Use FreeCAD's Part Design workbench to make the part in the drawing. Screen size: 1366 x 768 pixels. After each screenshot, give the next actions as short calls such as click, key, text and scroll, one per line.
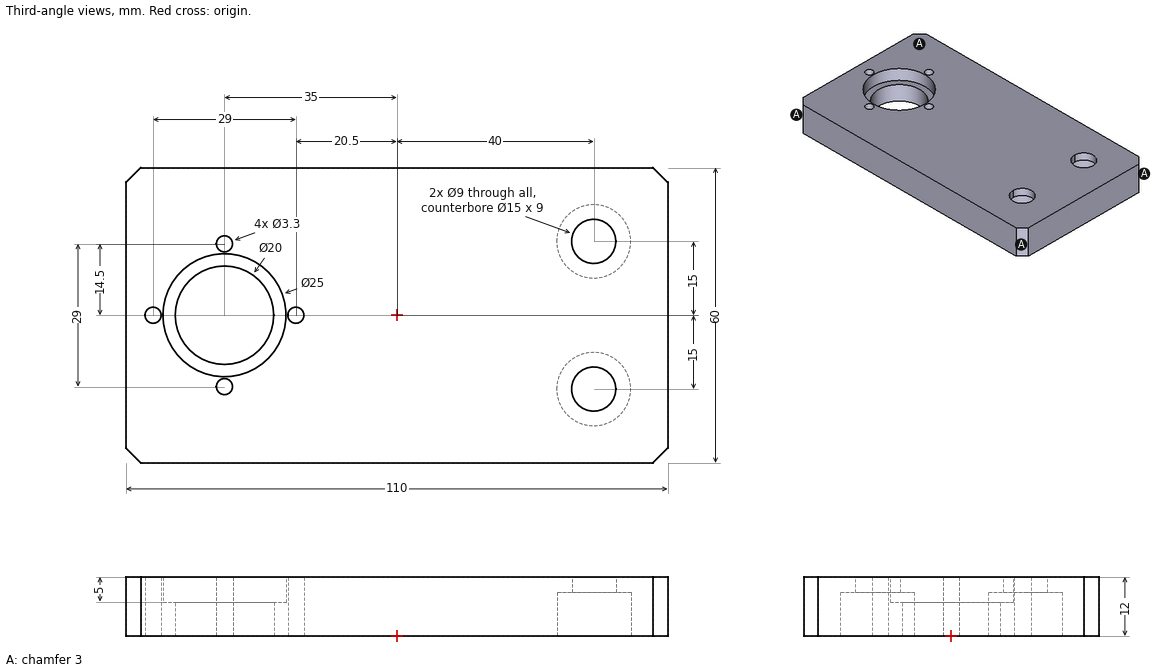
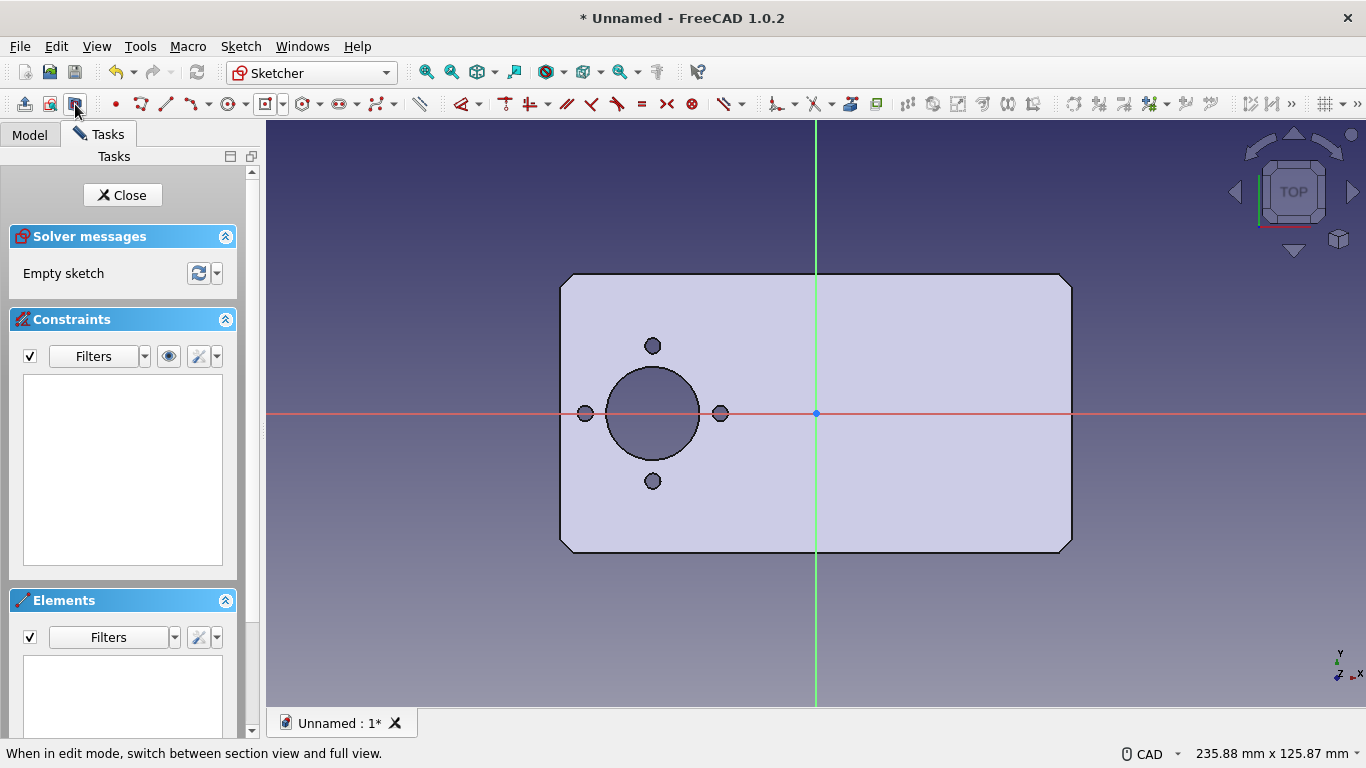
scroll(1060, 413, up, 4)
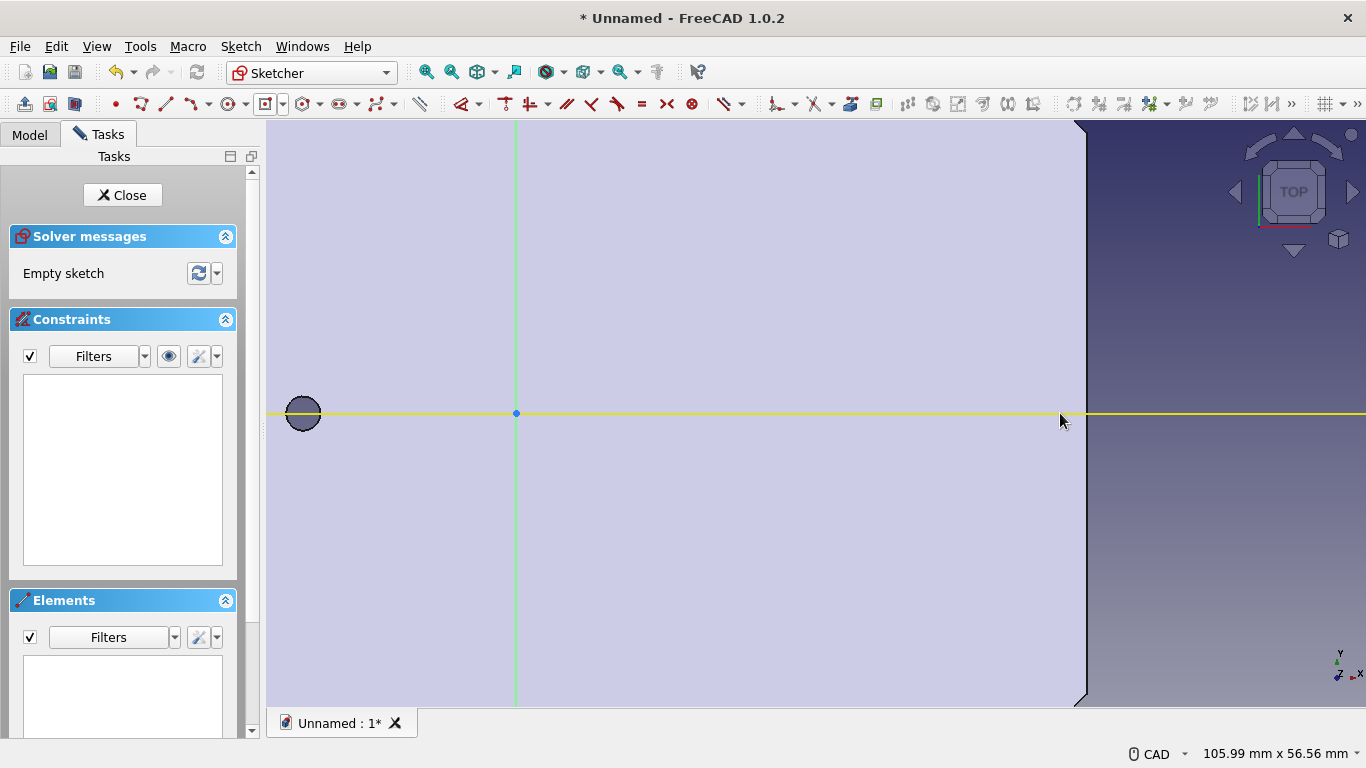
key(g)
key(c)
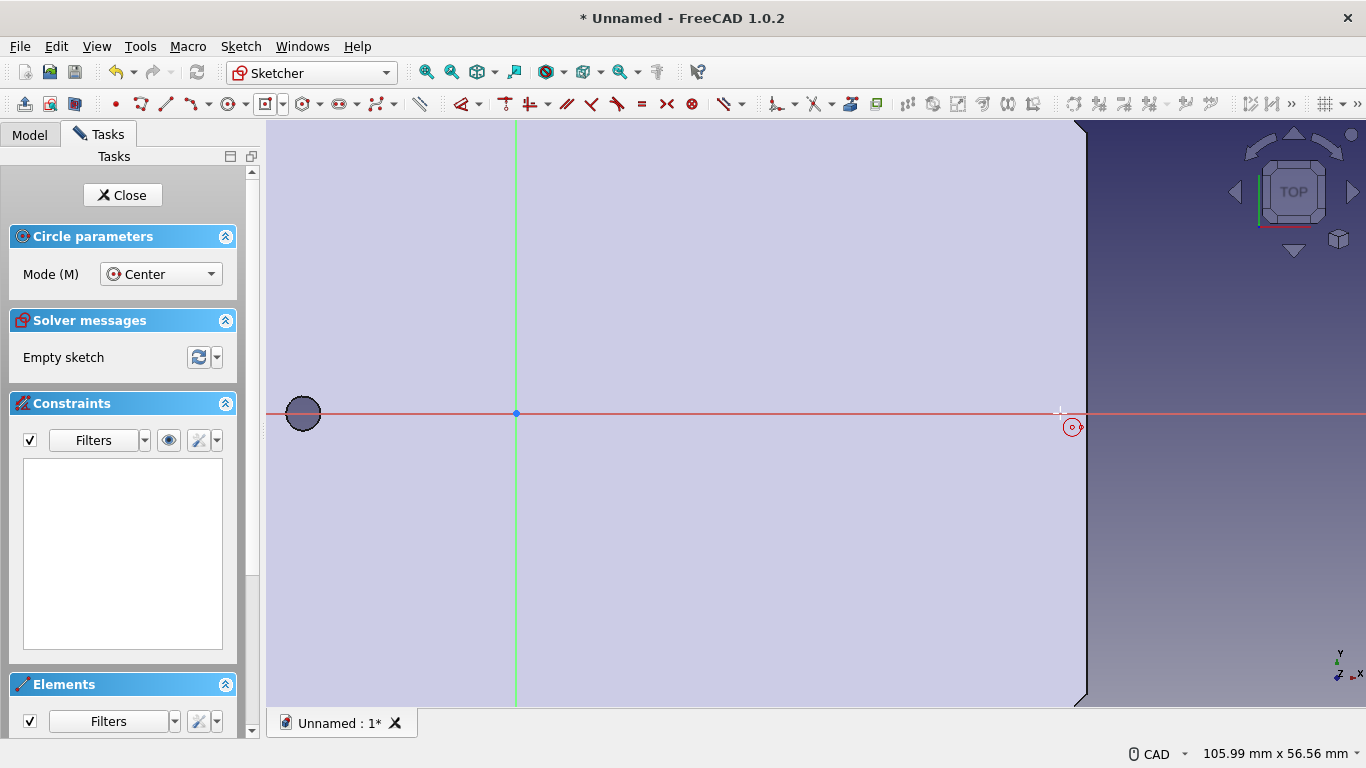
click(931, 258)
click(964, 225)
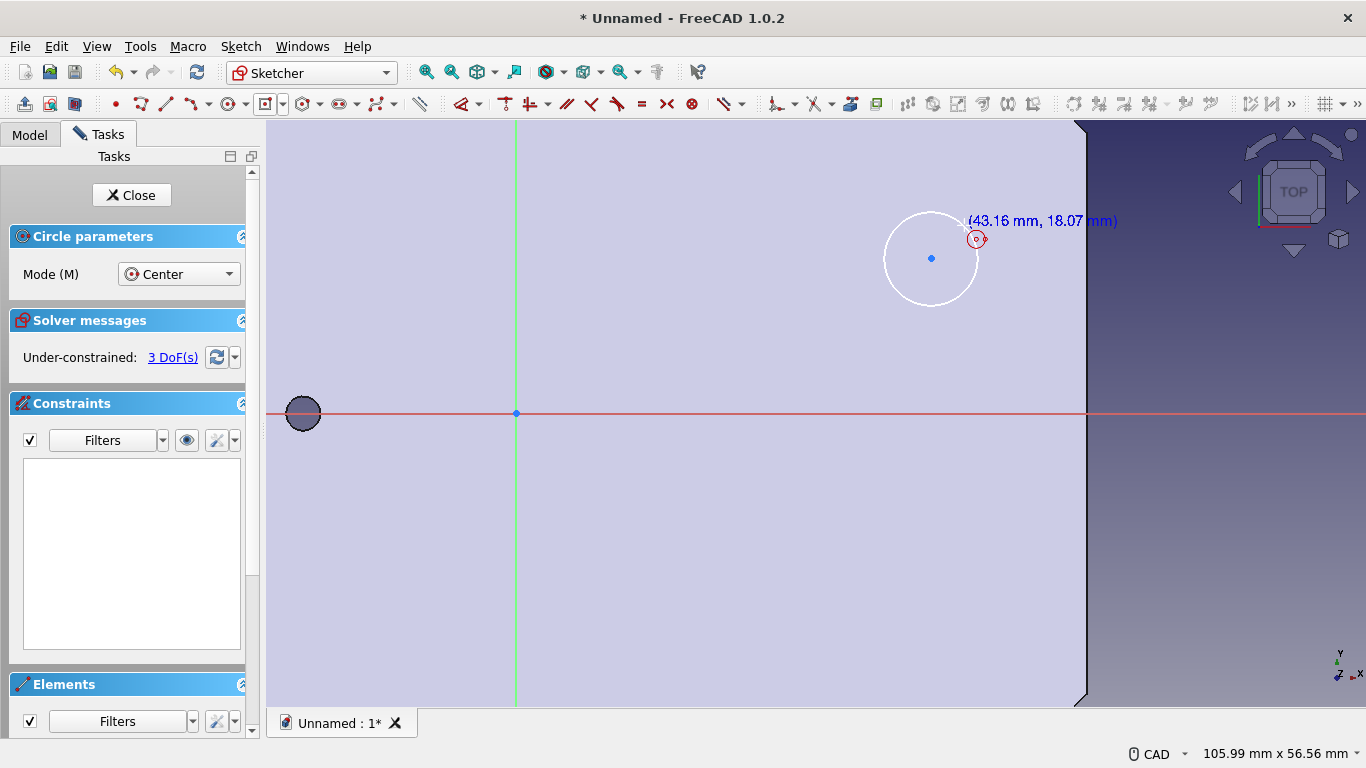
click(931, 569)
click(964, 536)
key(Escape)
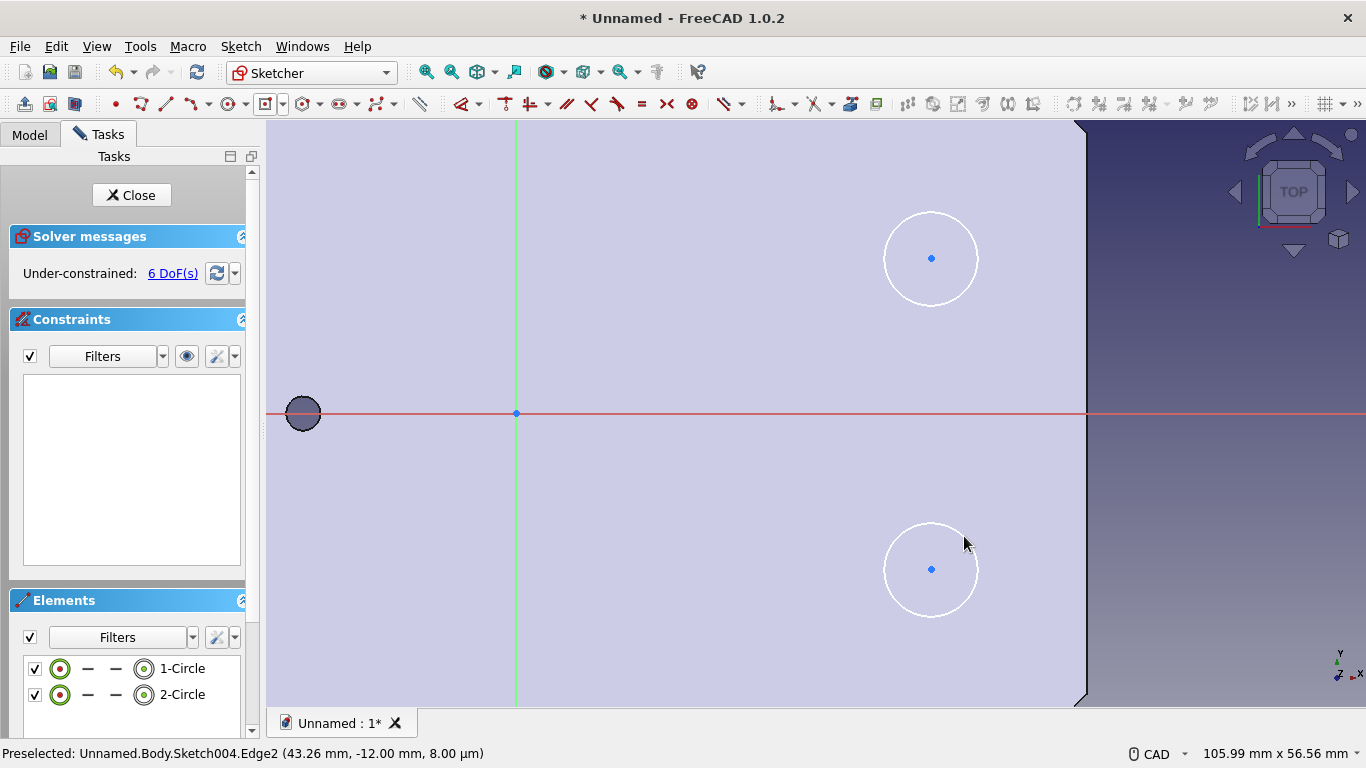
click(964, 226)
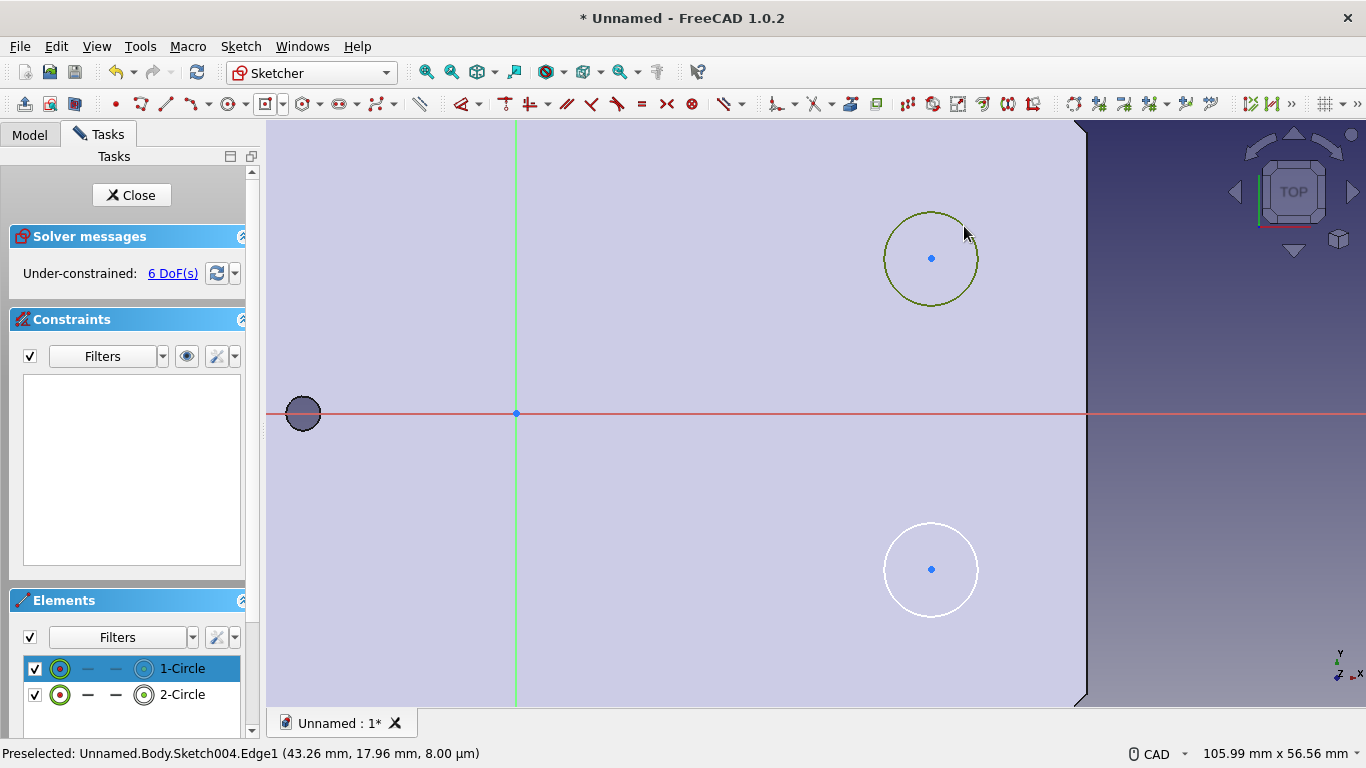
click(964, 537)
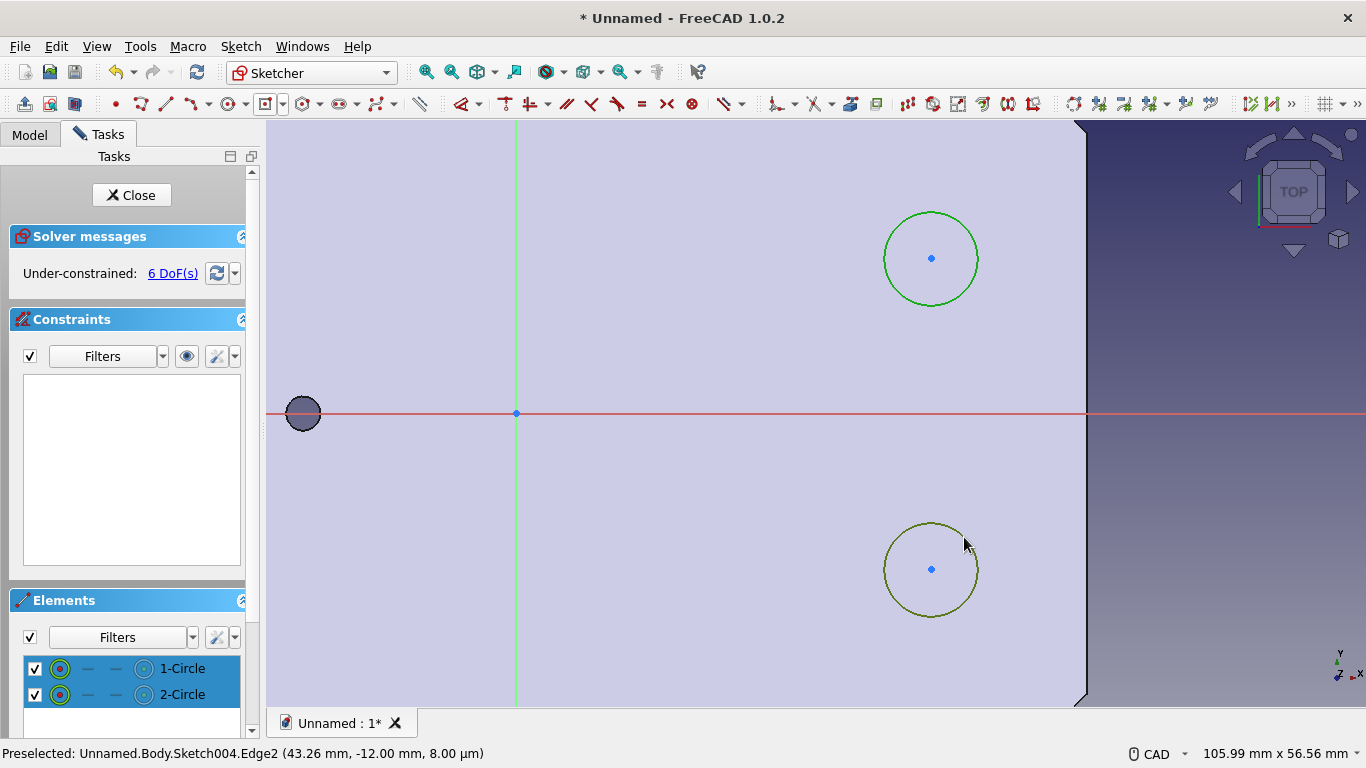
click(642, 104)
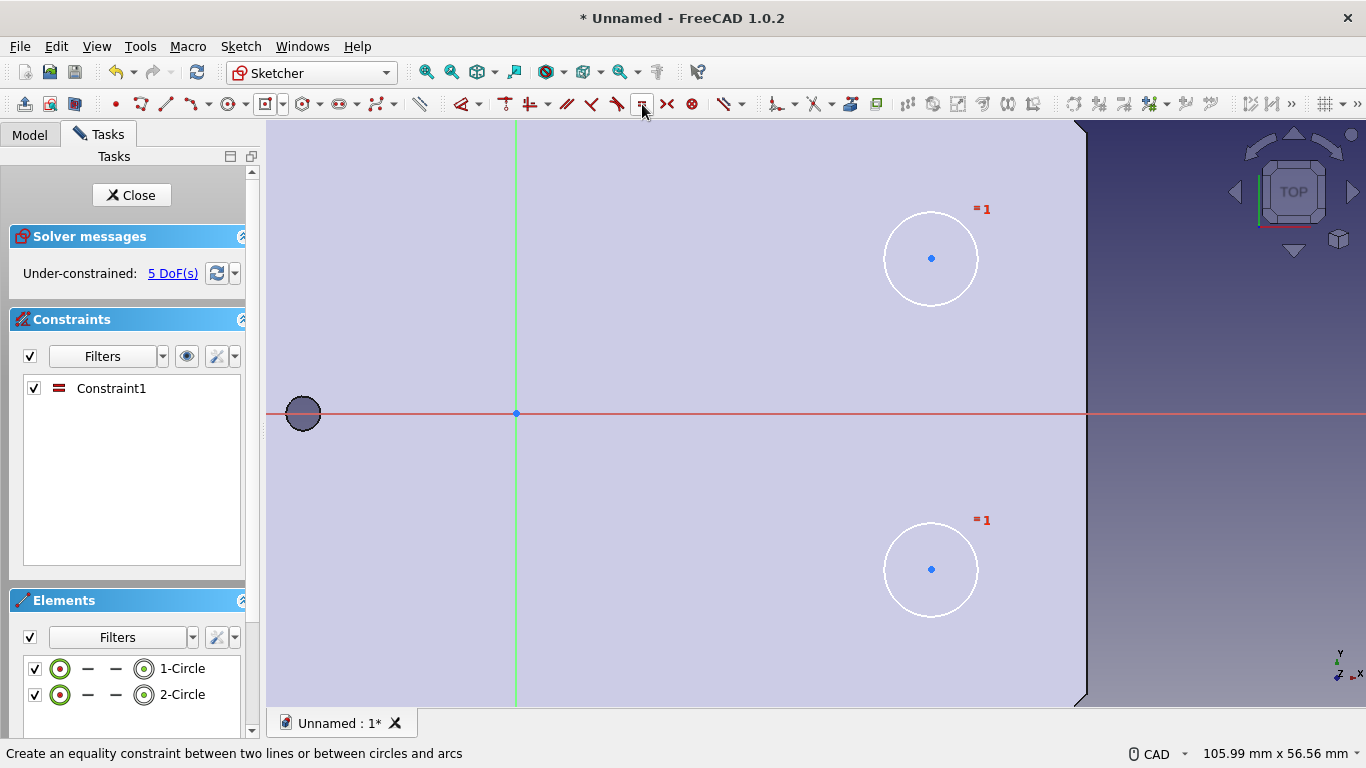
click(931, 259)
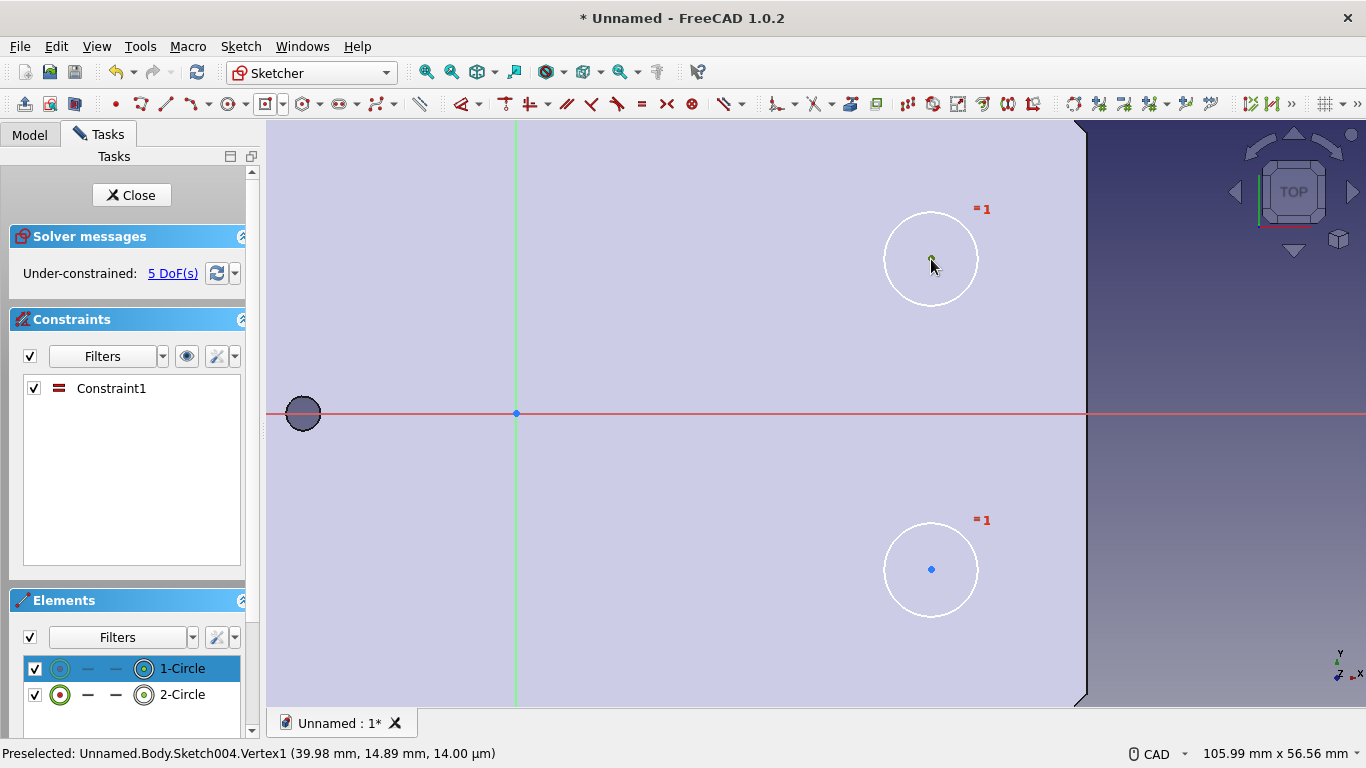
click(931, 570)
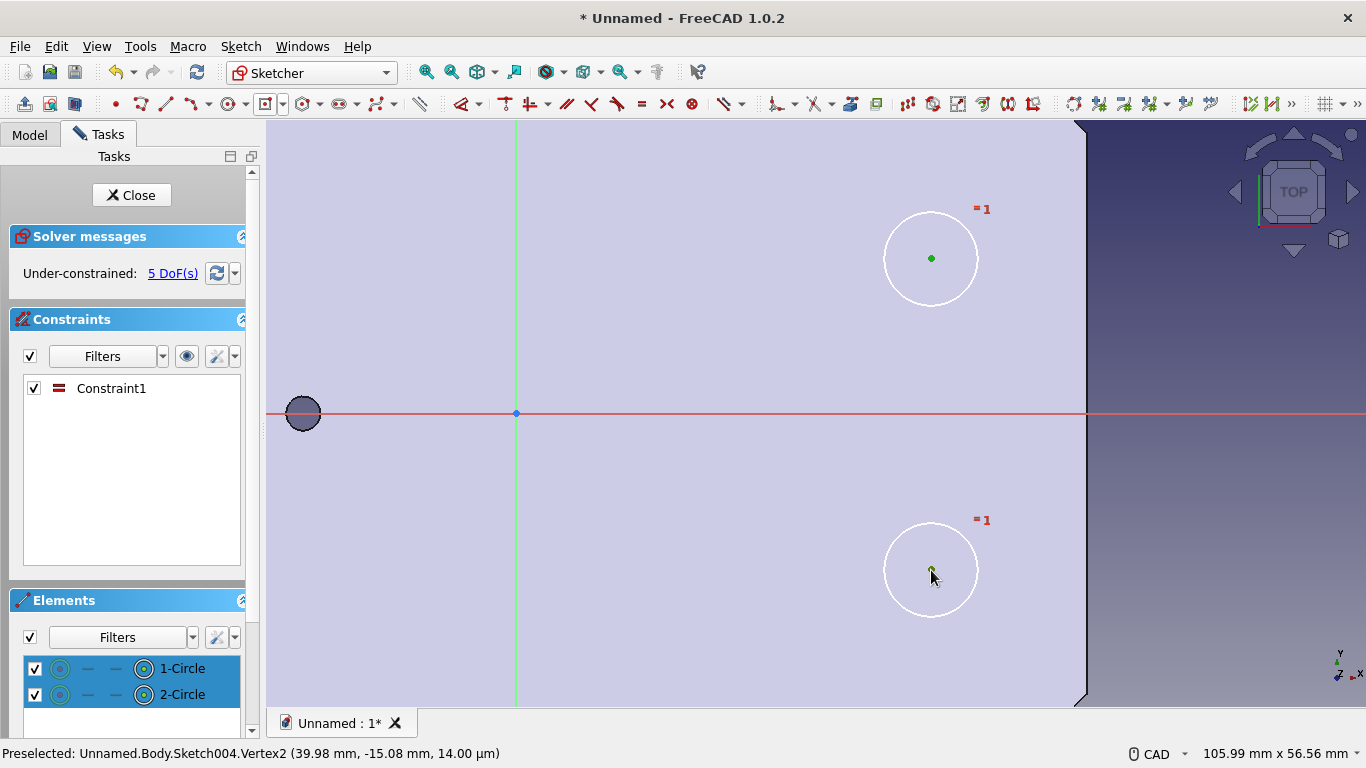
key(v)